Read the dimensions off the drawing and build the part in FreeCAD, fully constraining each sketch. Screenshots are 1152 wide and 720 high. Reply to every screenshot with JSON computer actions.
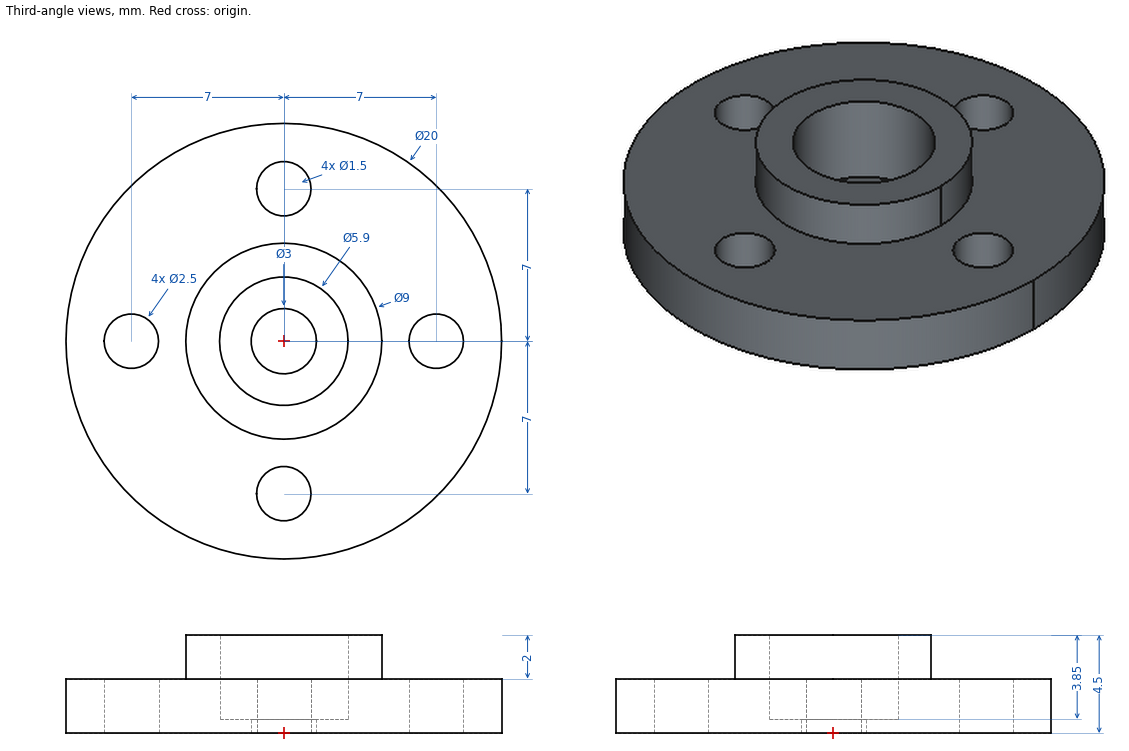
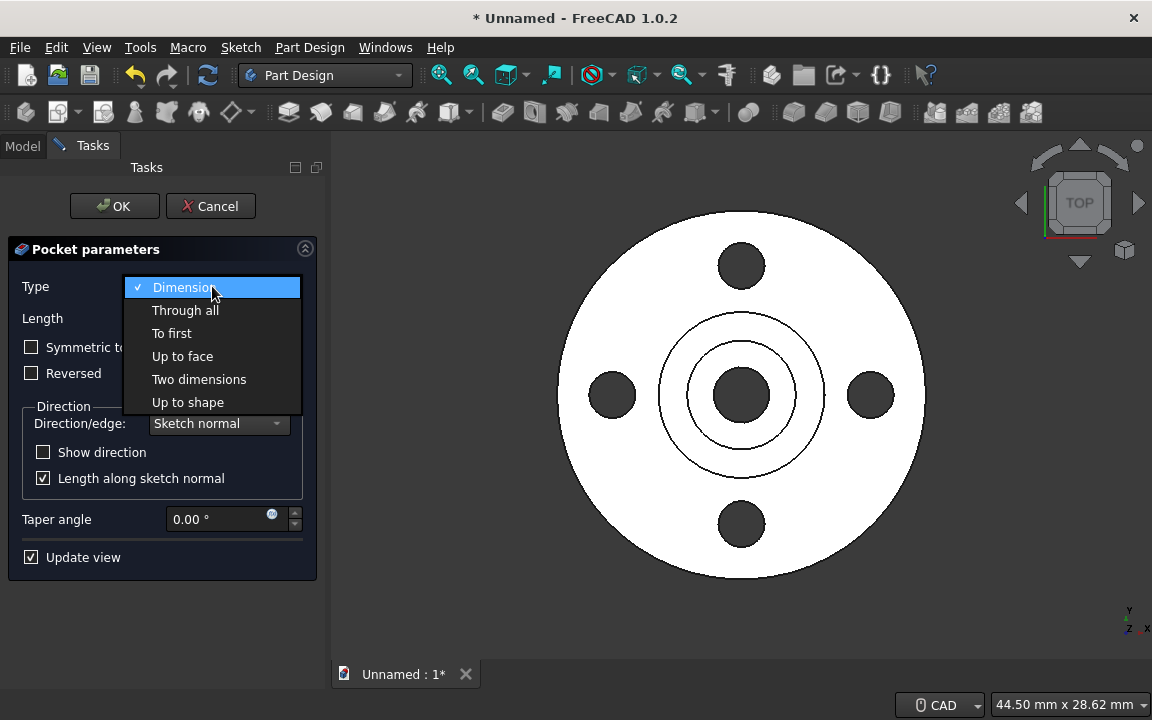
{"action": "left_click", "coordinate": [212, 310]}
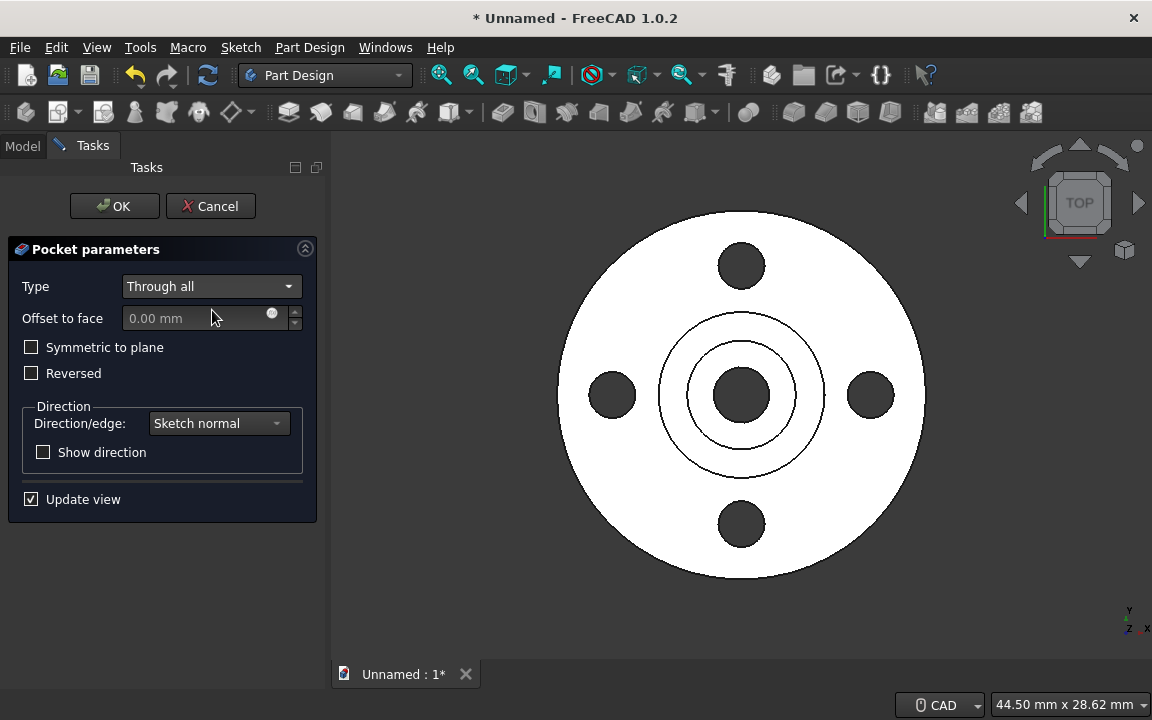
{"action": "left_click", "coordinate": [115, 206]}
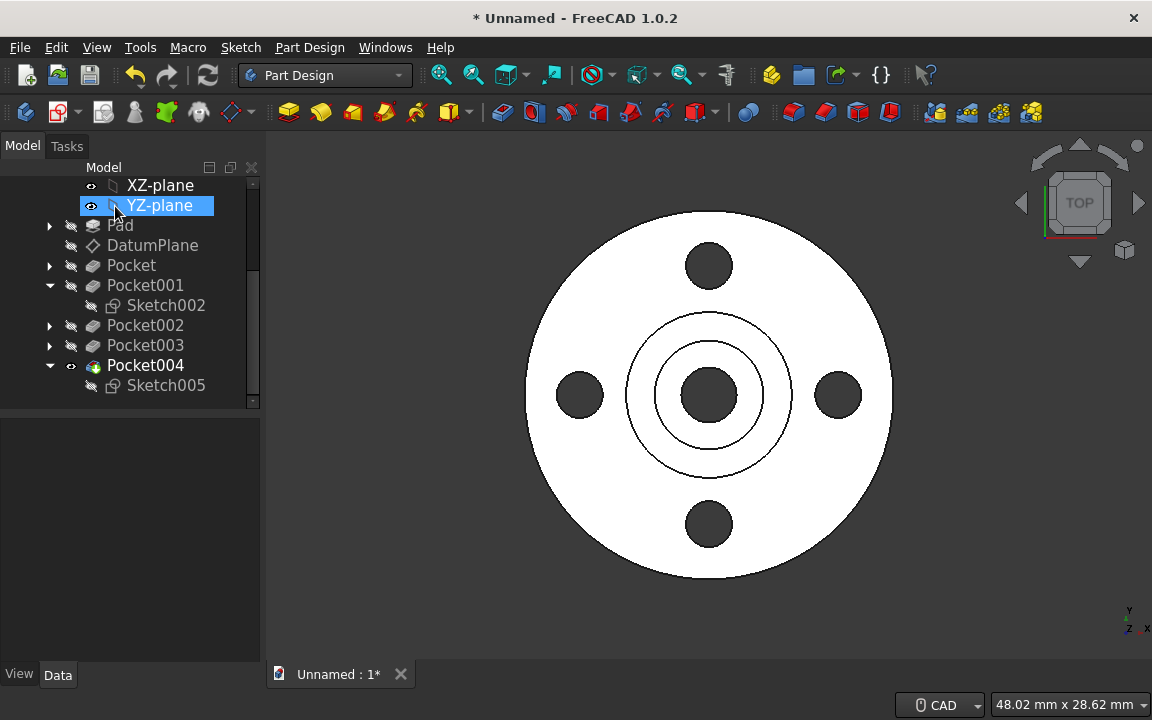
{"action": "key", "text": "0"}